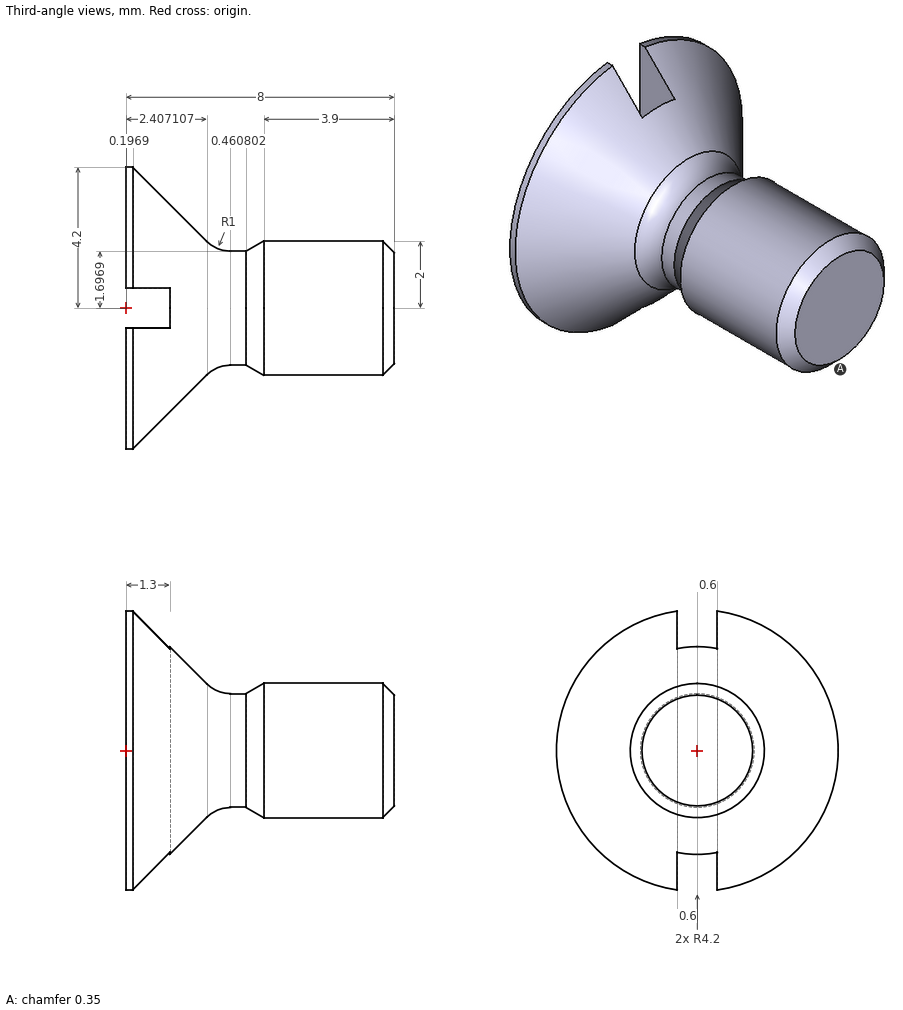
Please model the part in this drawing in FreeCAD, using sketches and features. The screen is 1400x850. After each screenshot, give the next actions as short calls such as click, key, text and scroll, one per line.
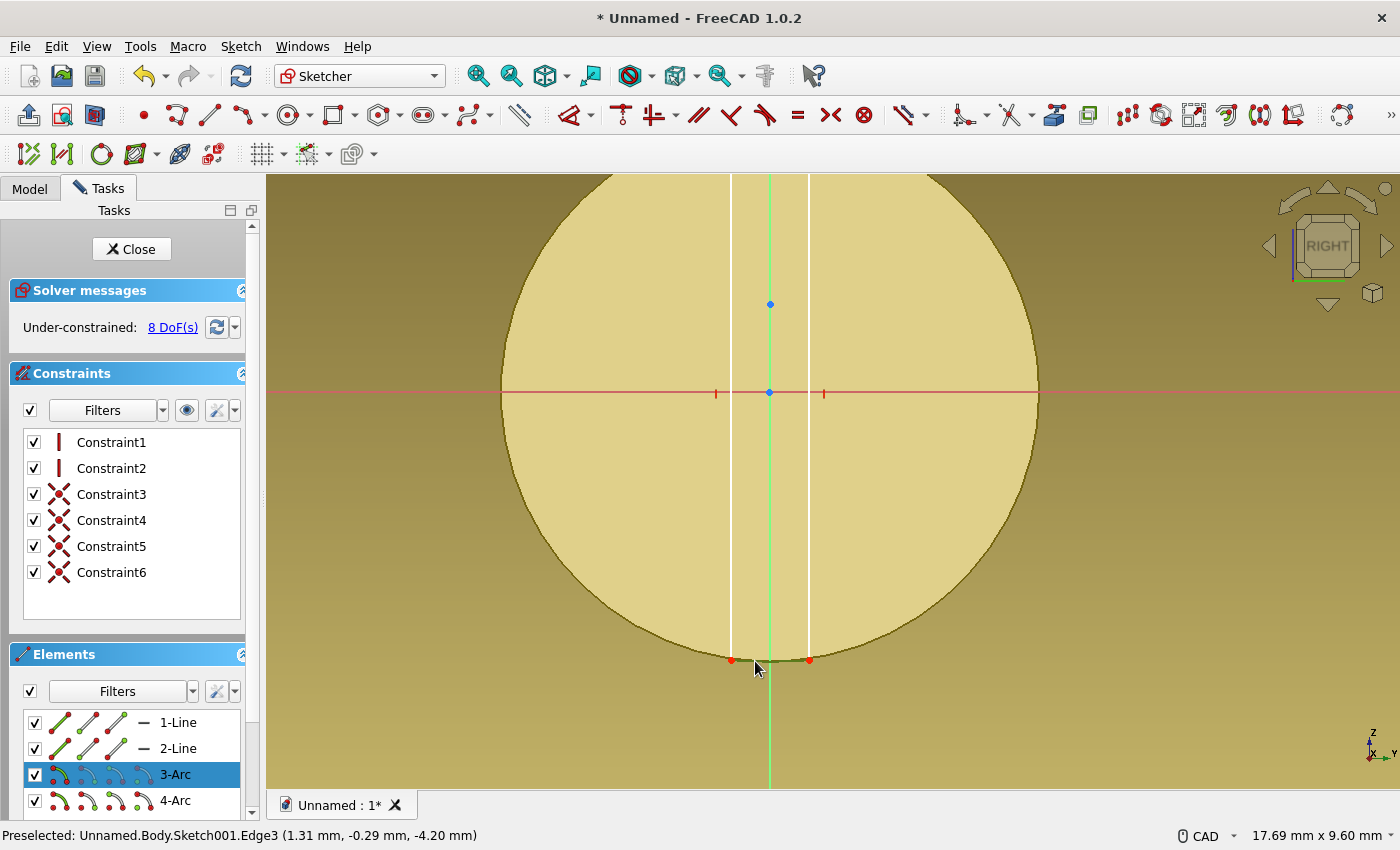
scroll(753, 663, down, 2)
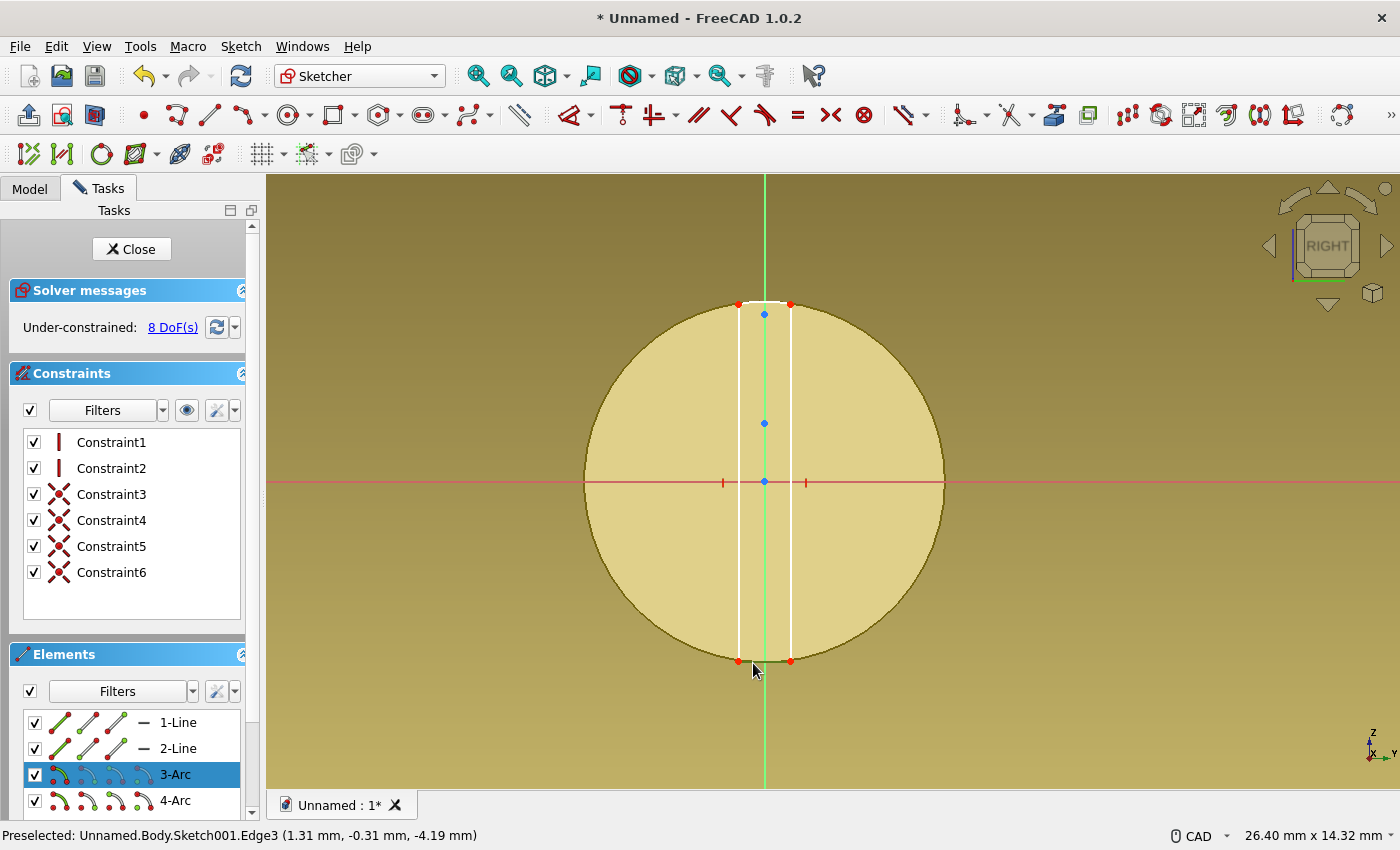
scroll(775, 302, up, 2)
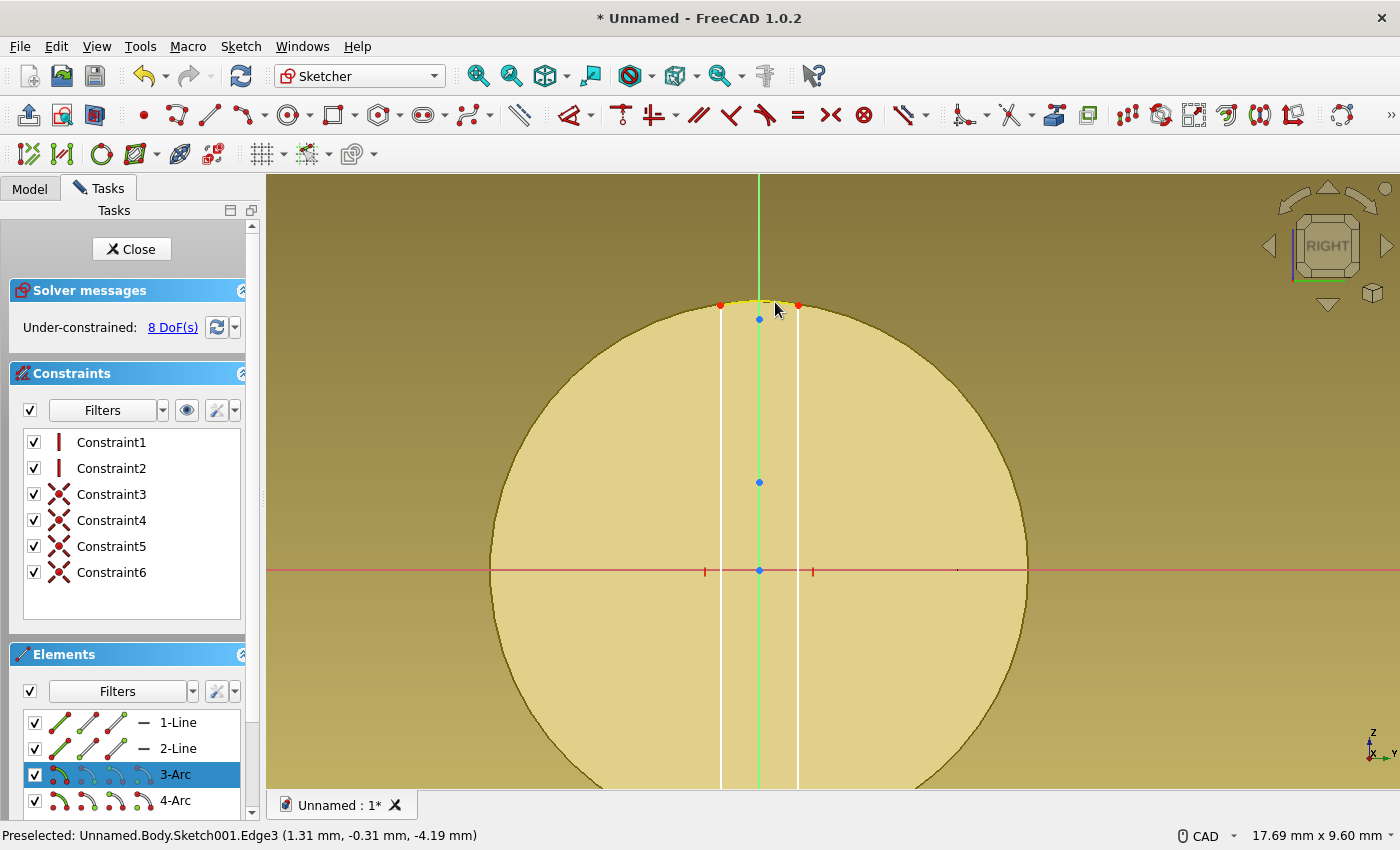
click(775, 302)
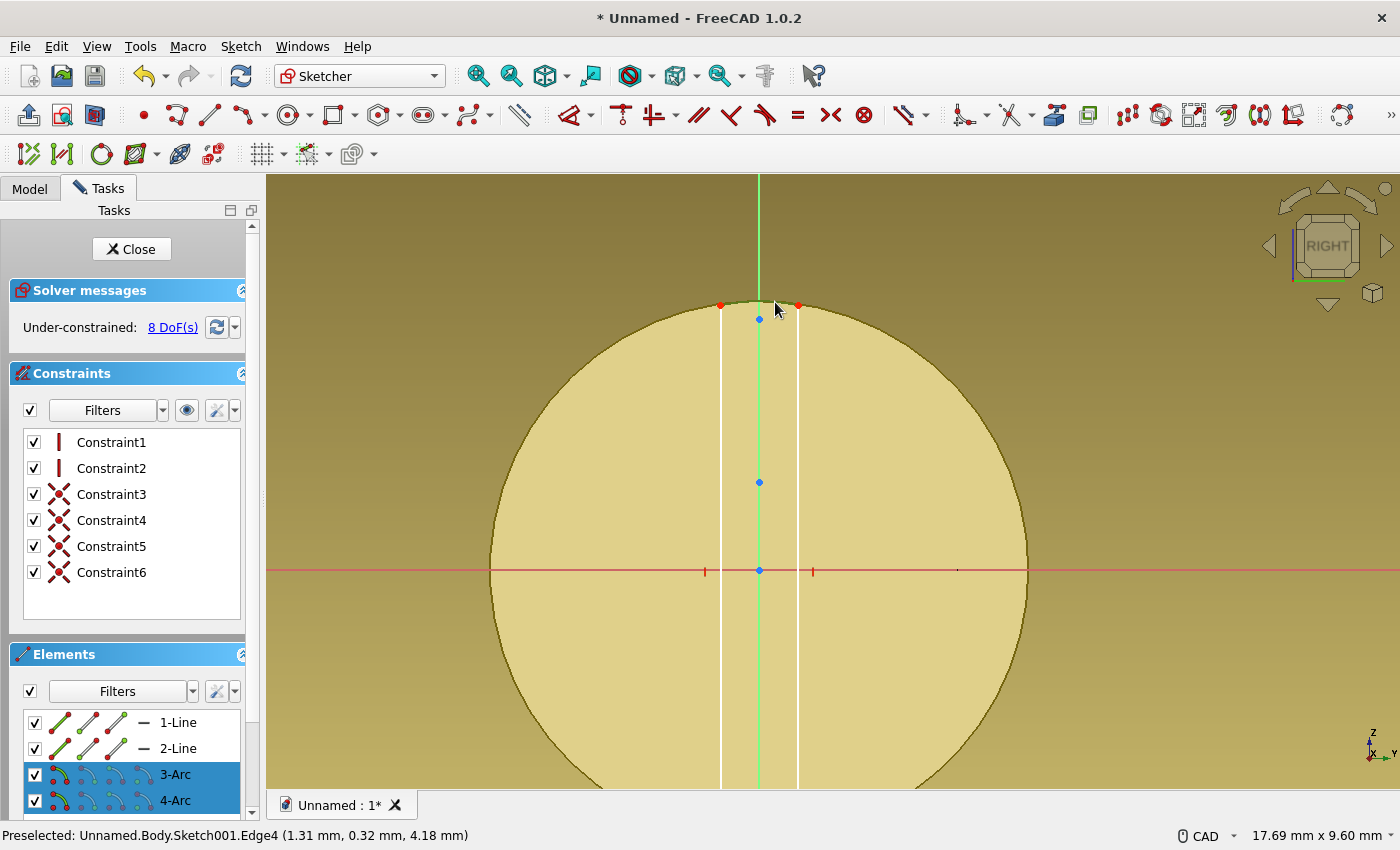
click(621, 116)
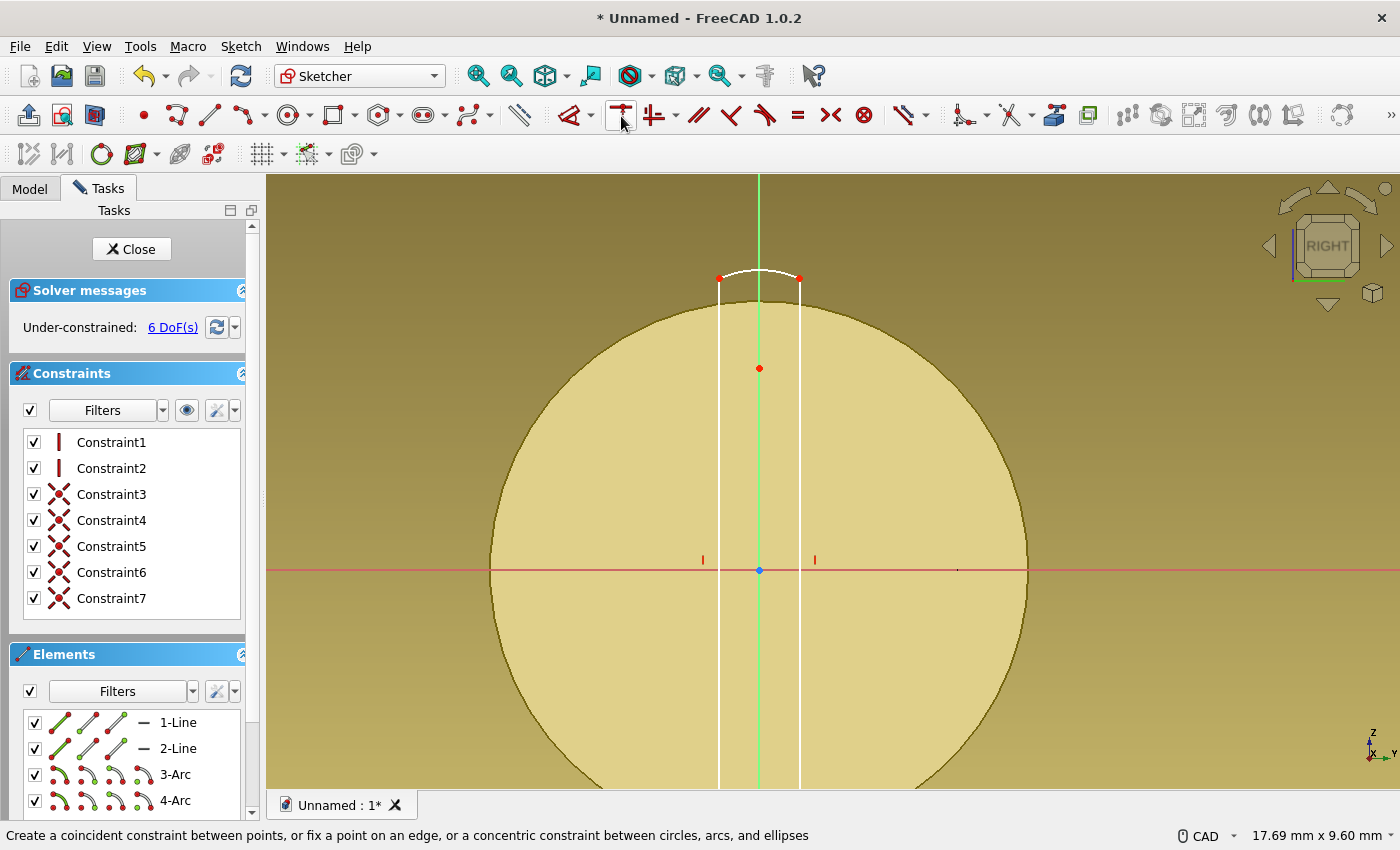
drag(749, 358, 769, 580)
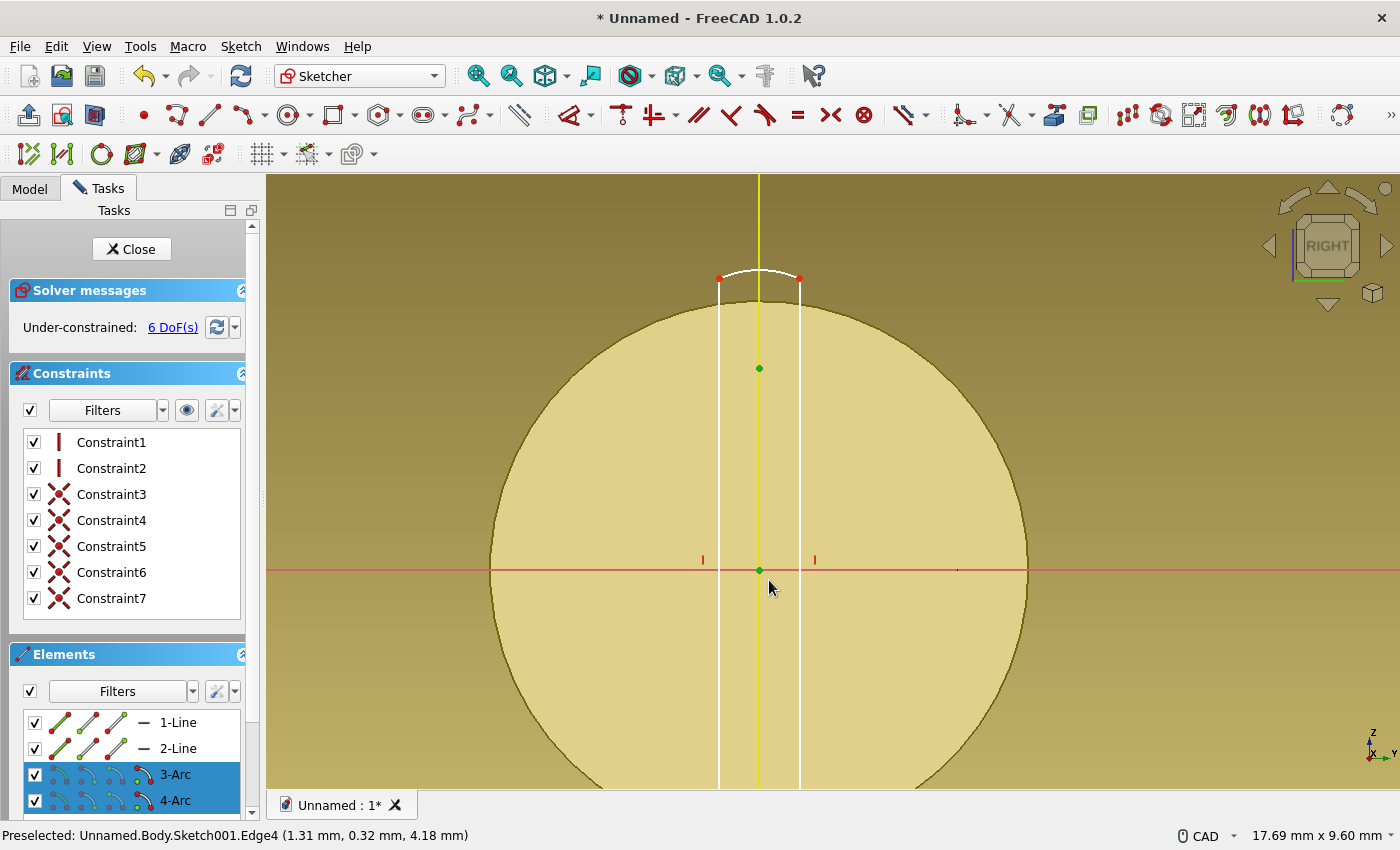
key(c)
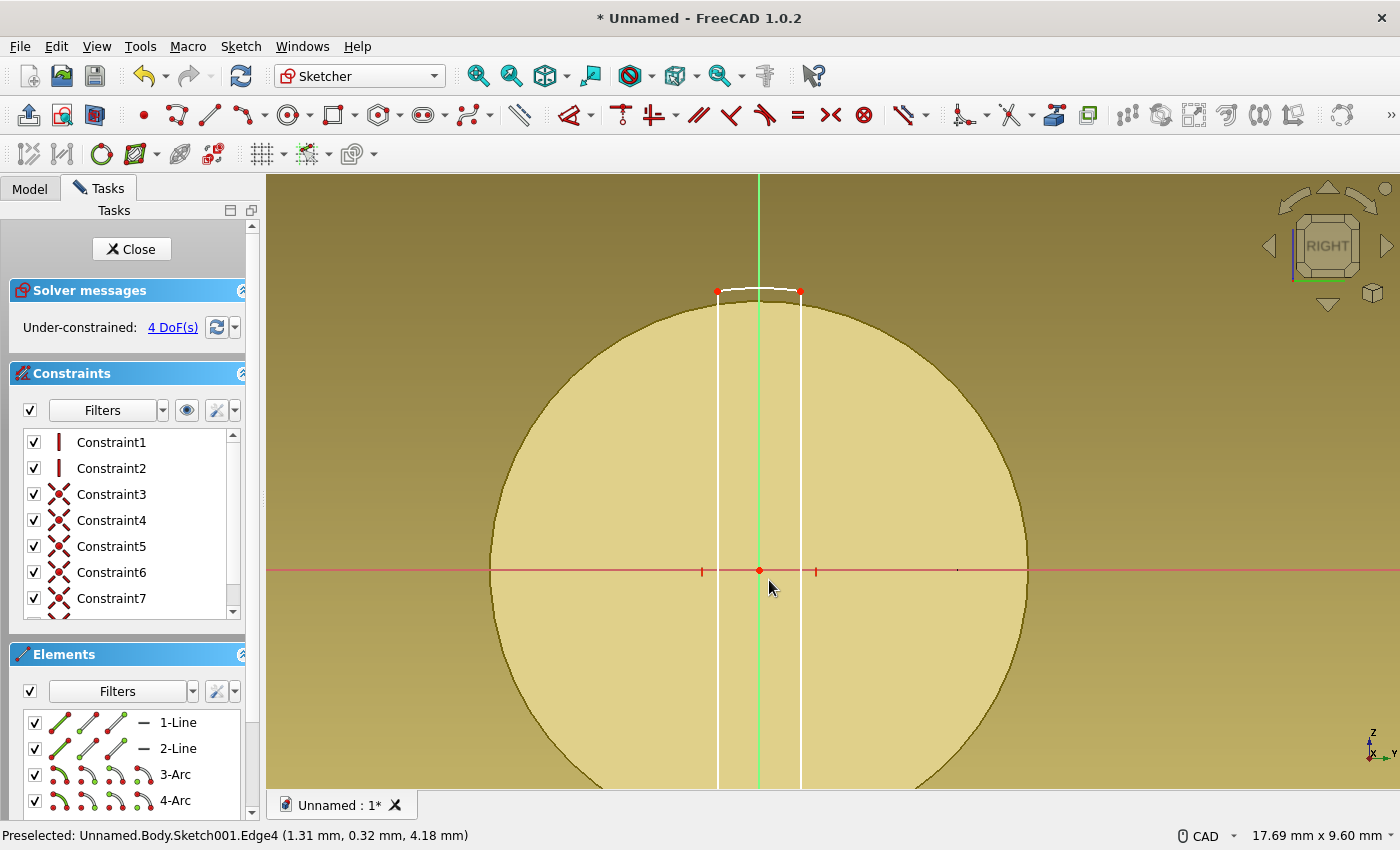
scroll(775, 301, down, 2)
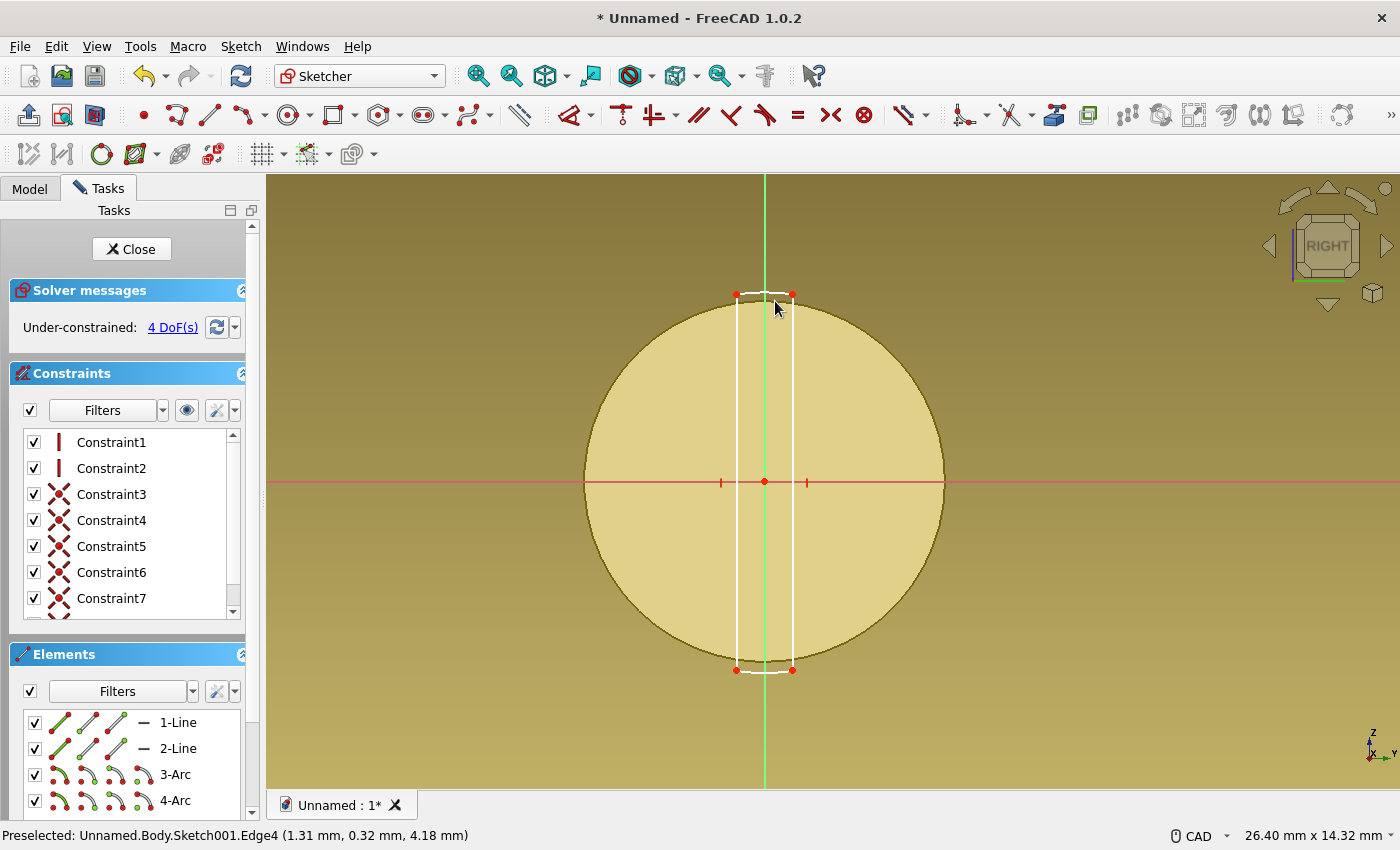
scroll(754, 673, up, 2)